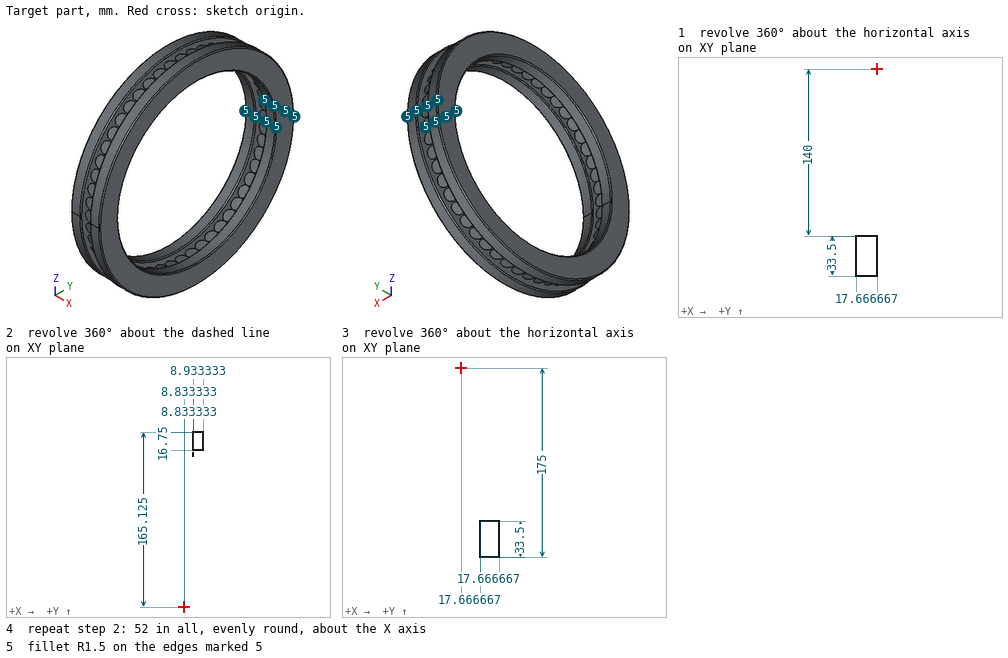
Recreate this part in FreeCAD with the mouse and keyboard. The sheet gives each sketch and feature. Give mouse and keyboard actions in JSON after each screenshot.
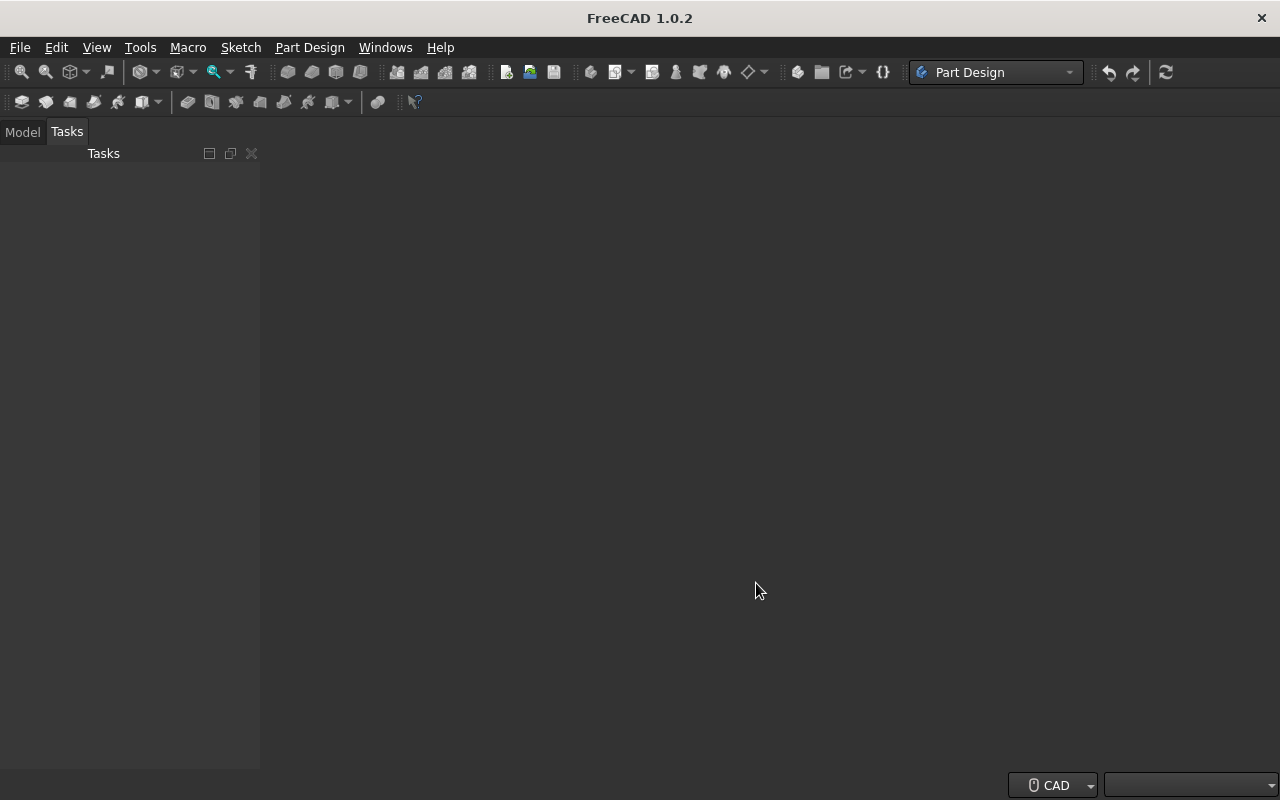
{"action": "left_click", "coordinate": [506, 72]}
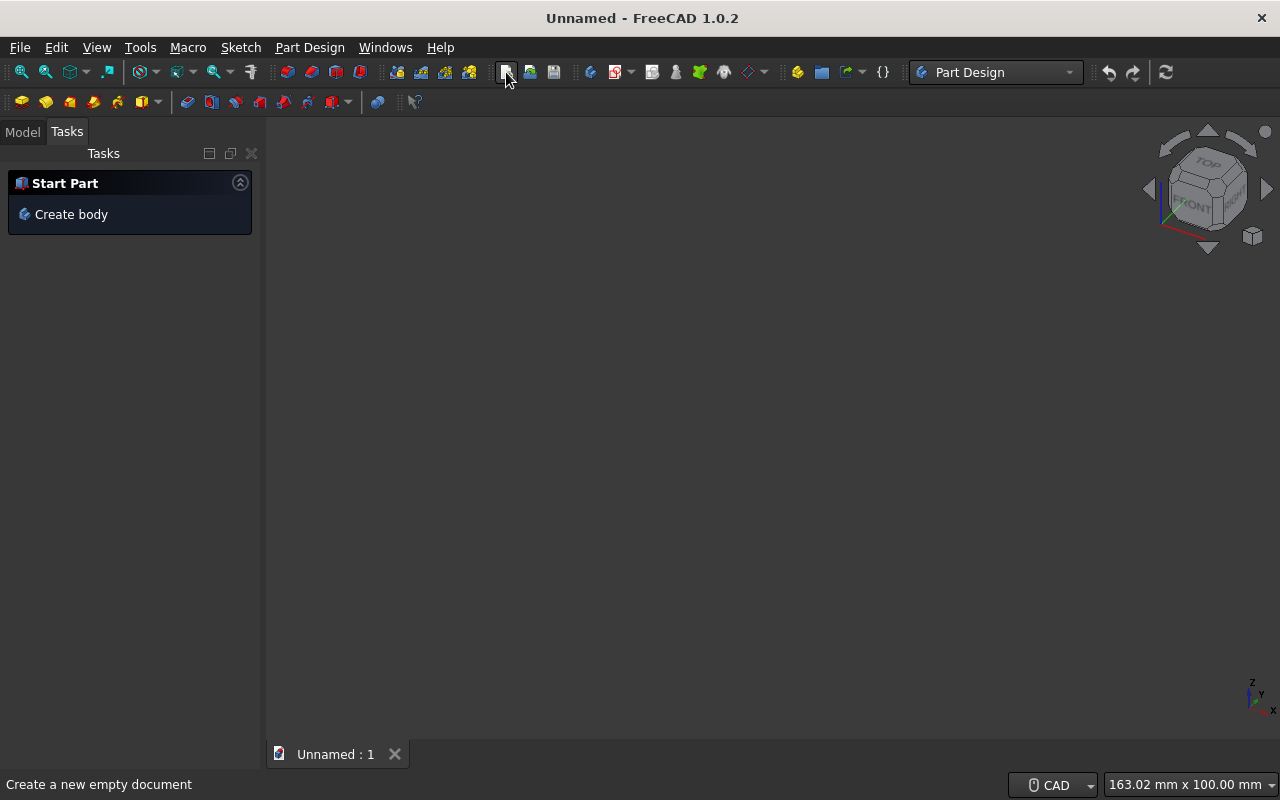
{"action": "left_click", "coordinate": [616, 72]}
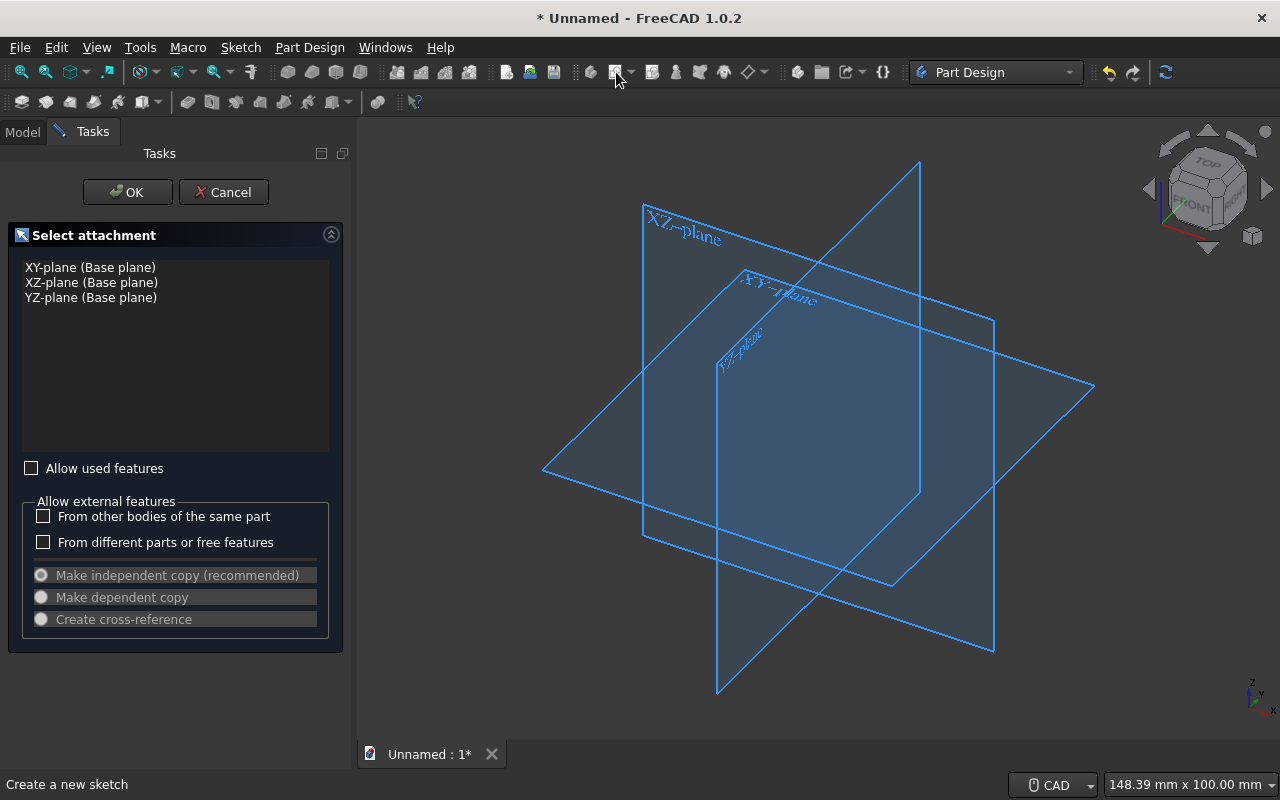
{"action": "left_click", "coordinate": [82, 268]}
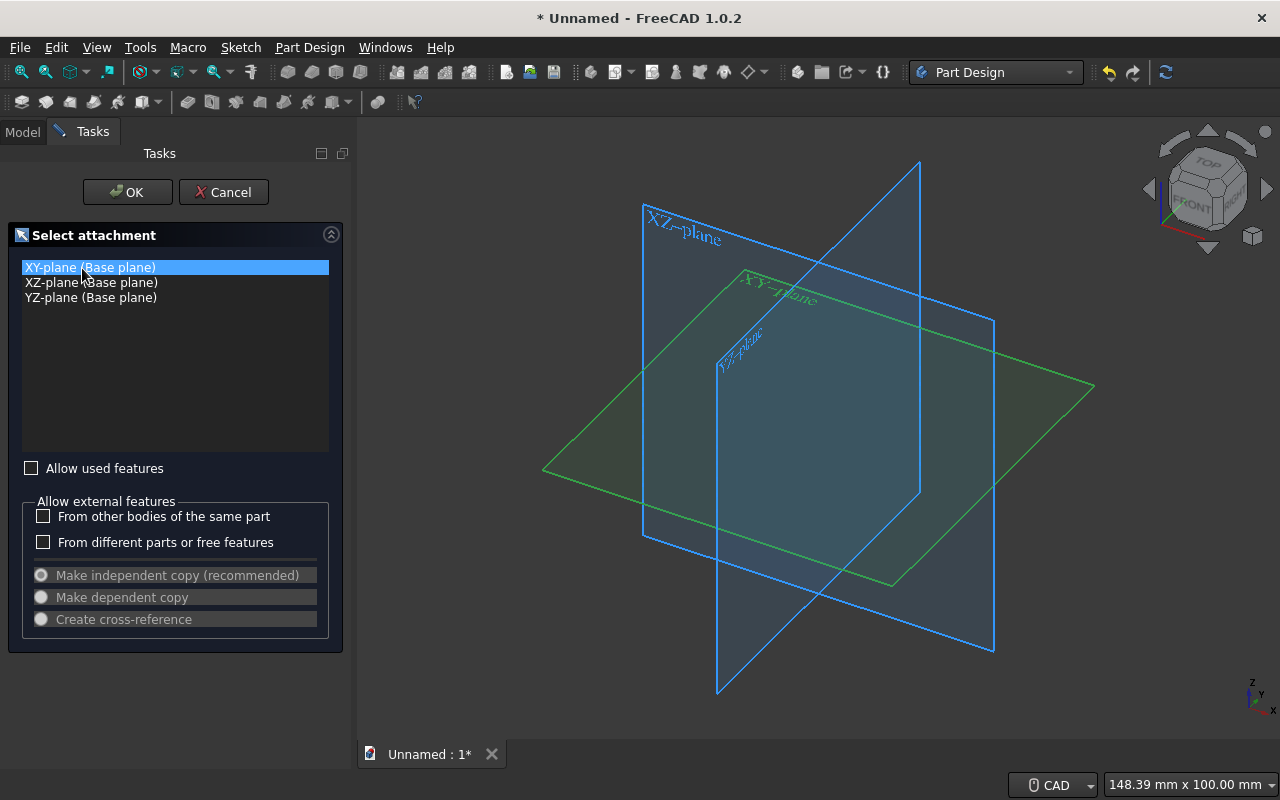
{"action": "left_click", "coordinate": [128, 192]}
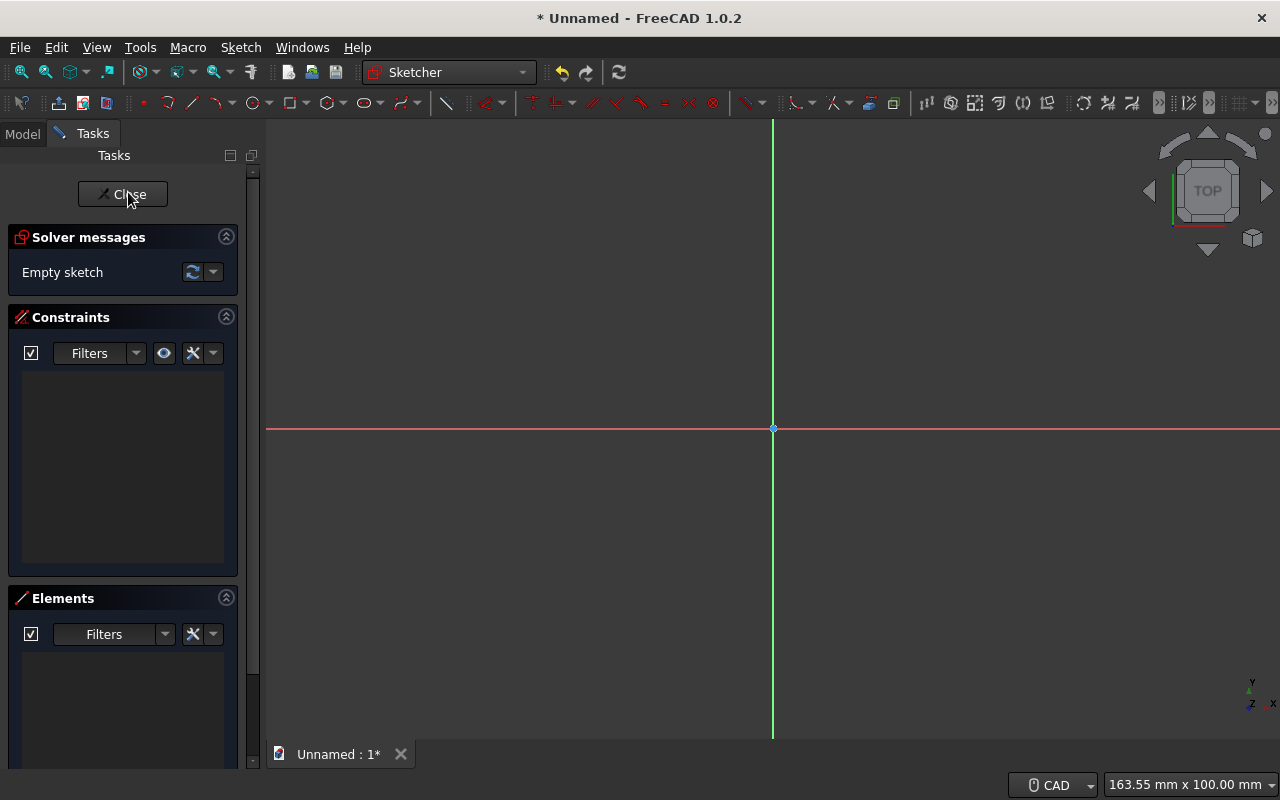
{"action": "scroll", "coordinate": [704, 429], "scroll_direction": "down", "scroll_amount": 5}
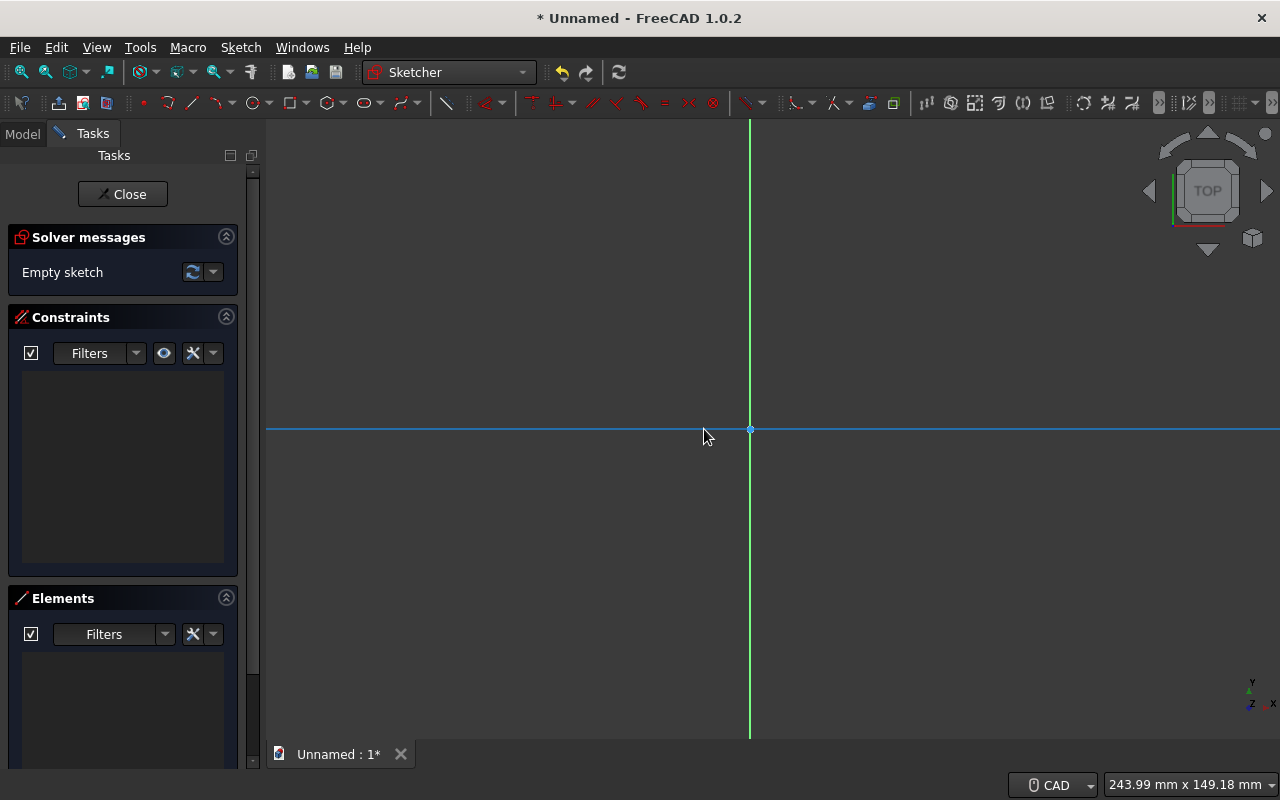
{"action": "scroll", "coordinate": [704, 429], "scroll_direction": "down", "scroll_amount": 5}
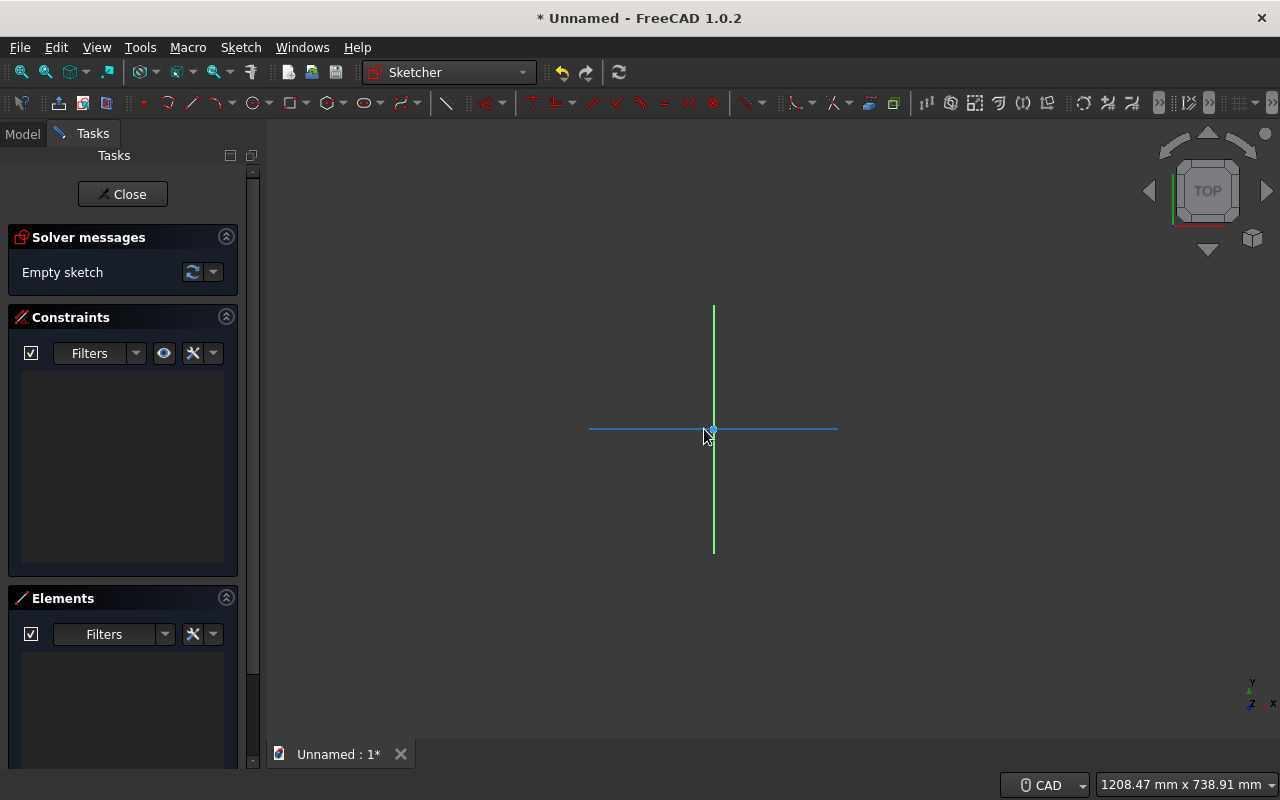
{"action": "scroll", "coordinate": [706, 572], "scroll_direction": "up", "scroll_amount": 13}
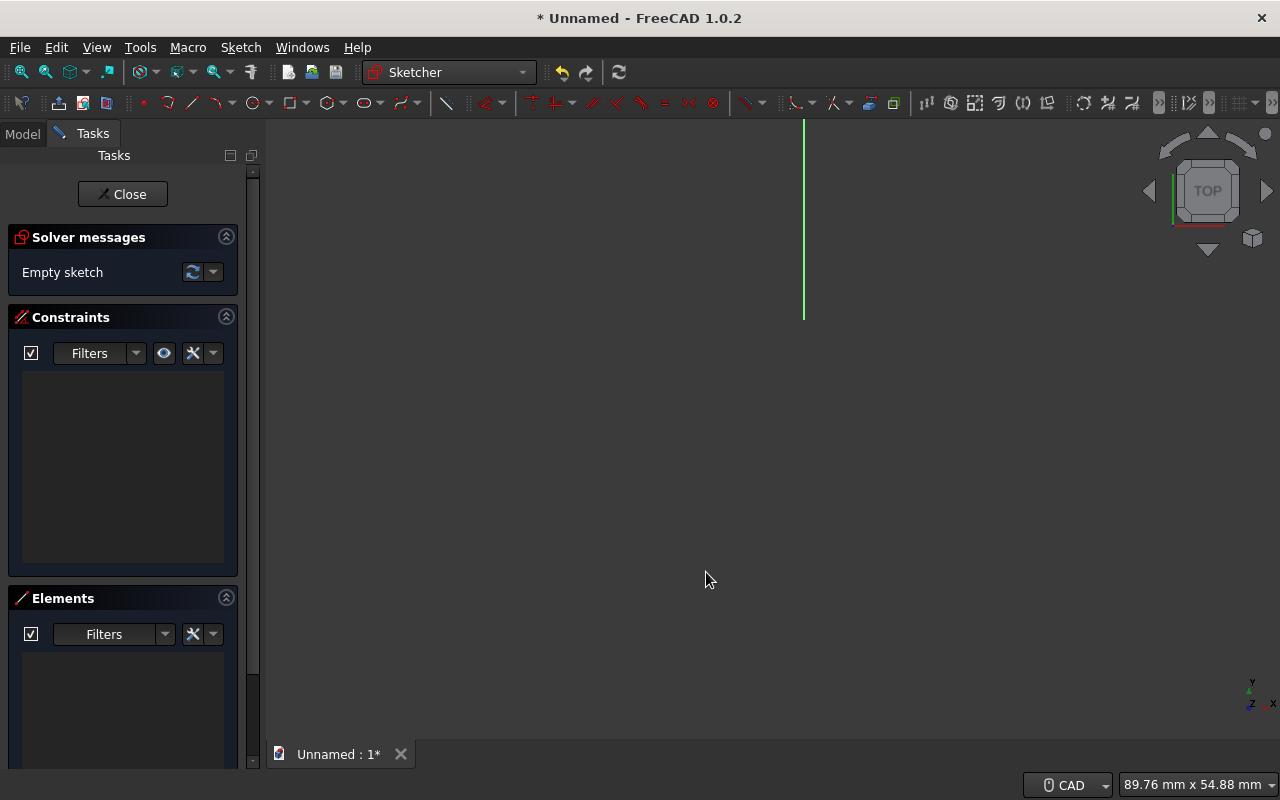
{"action": "left_click", "coordinate": [290, 104]}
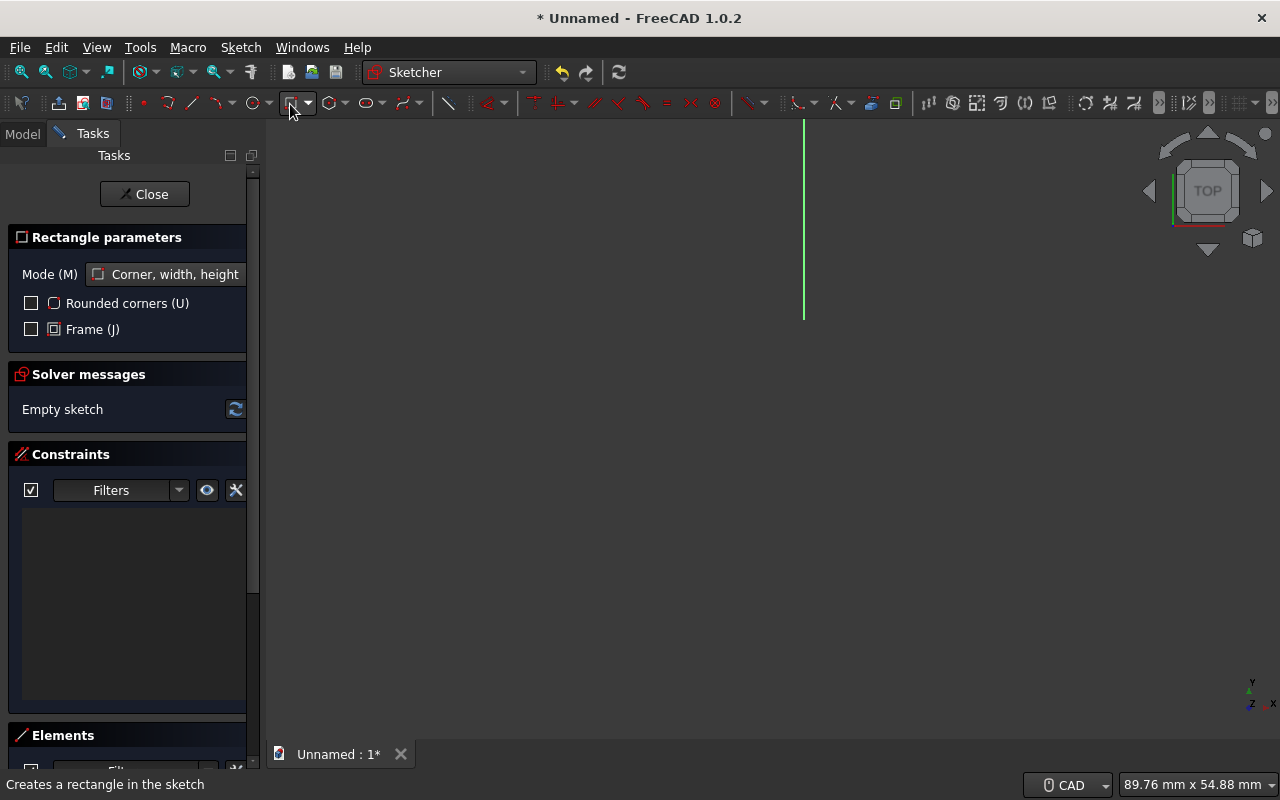
{"action": "left_click", "coordinate": [605, 225]}
{"action": "left_click", "coordinate": [804, 603]}
{"action": "key", "text": "Escape"}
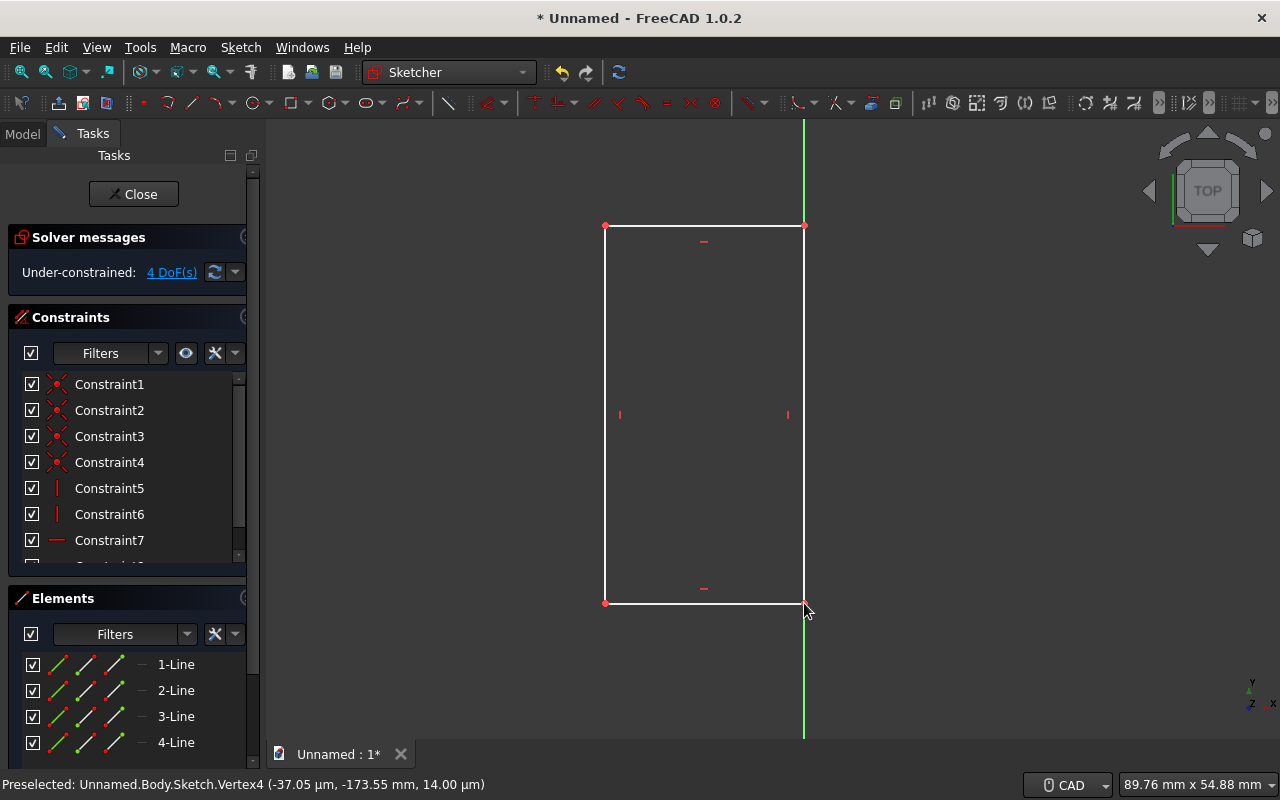
{"action": "left_click", "coordinate": [804, 604]}